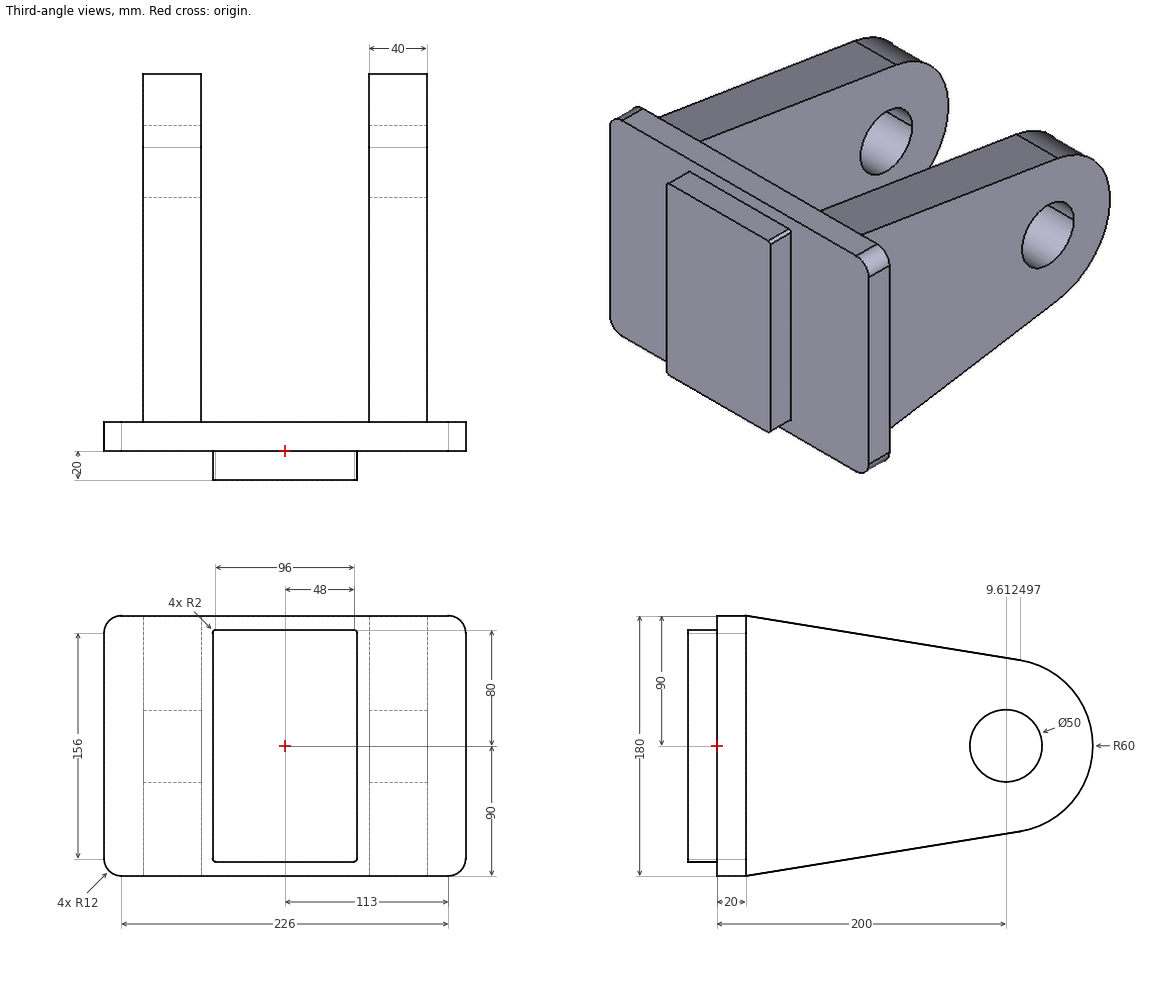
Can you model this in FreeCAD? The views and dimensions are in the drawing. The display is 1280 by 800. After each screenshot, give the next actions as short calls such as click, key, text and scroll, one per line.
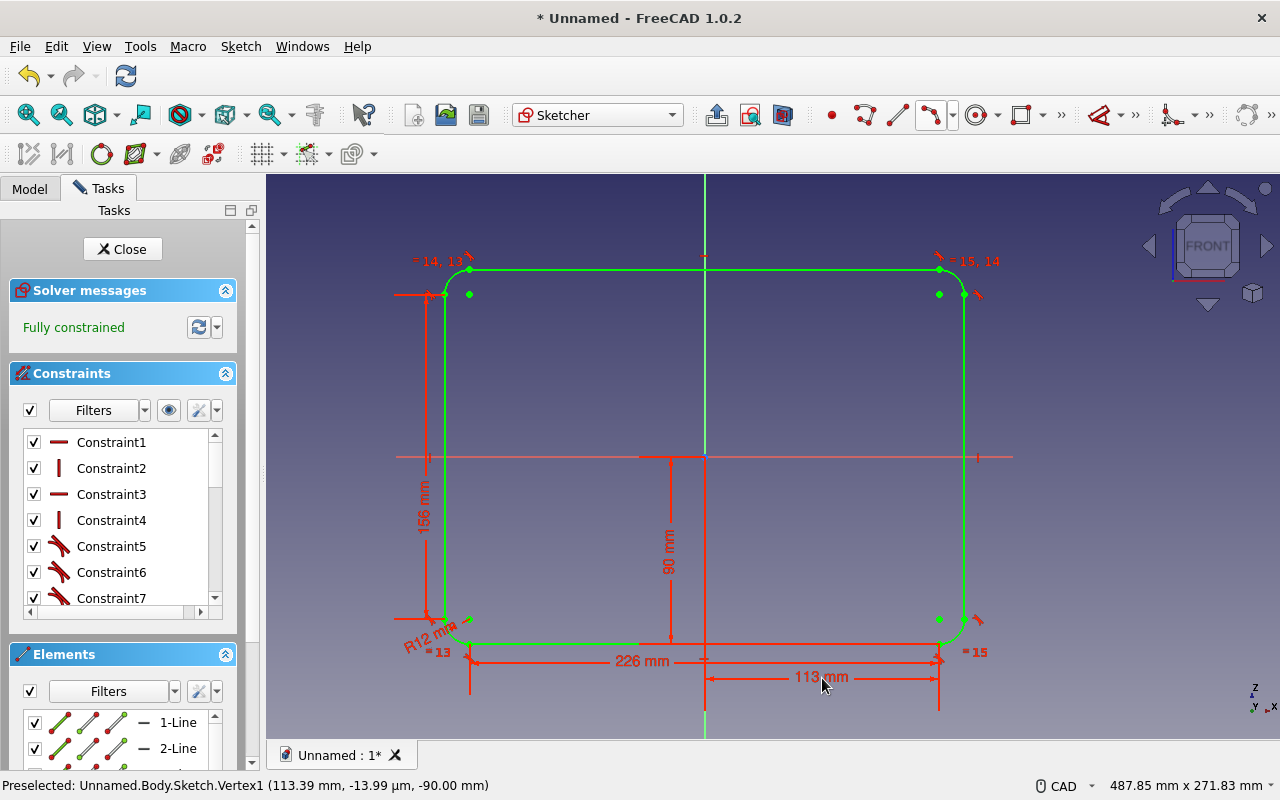
click(123, 249)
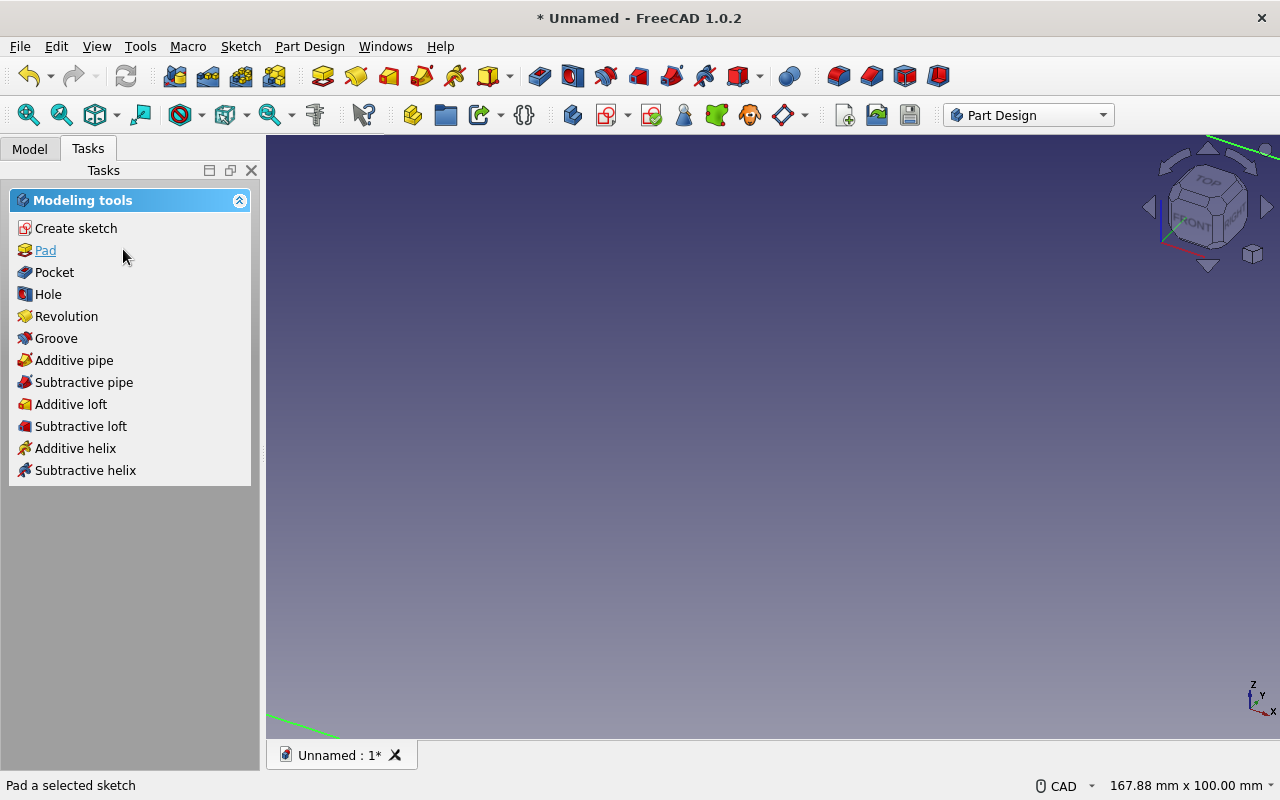
click(323, 76)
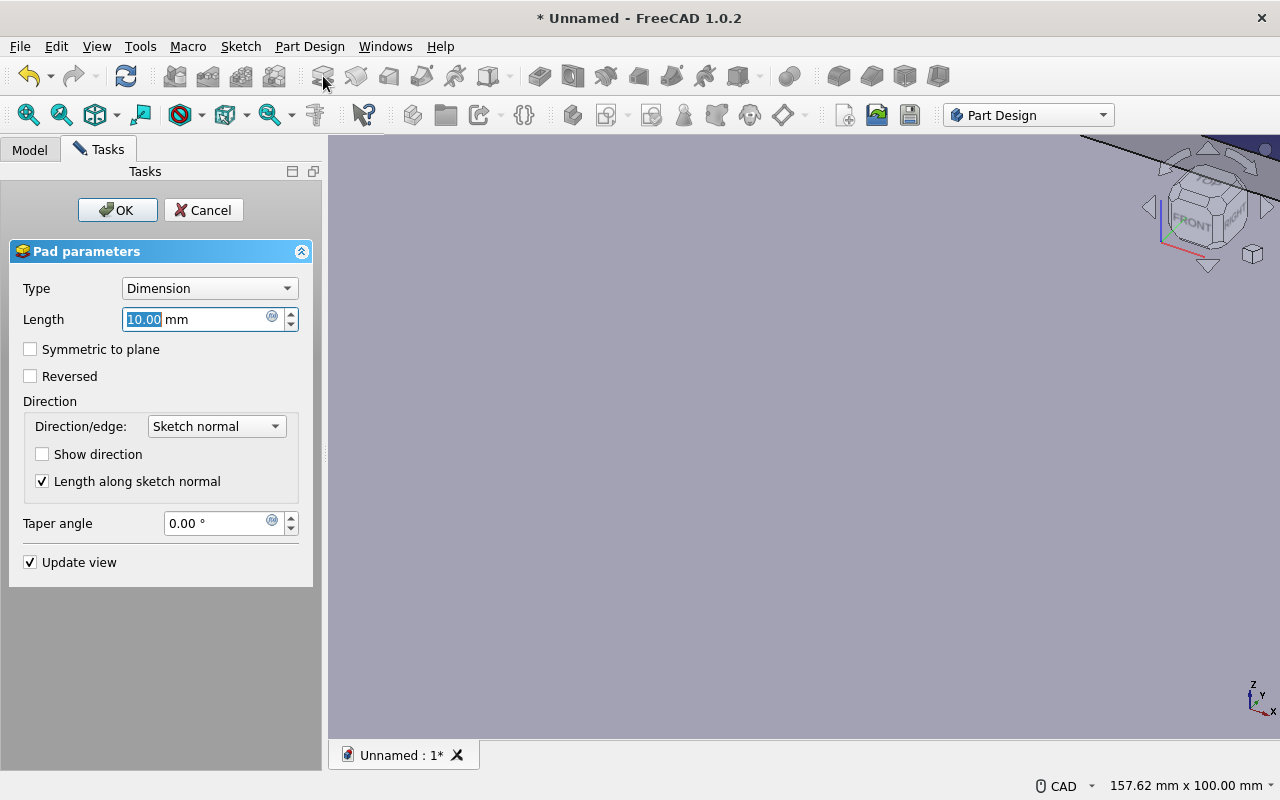
text(20)
key(Tab)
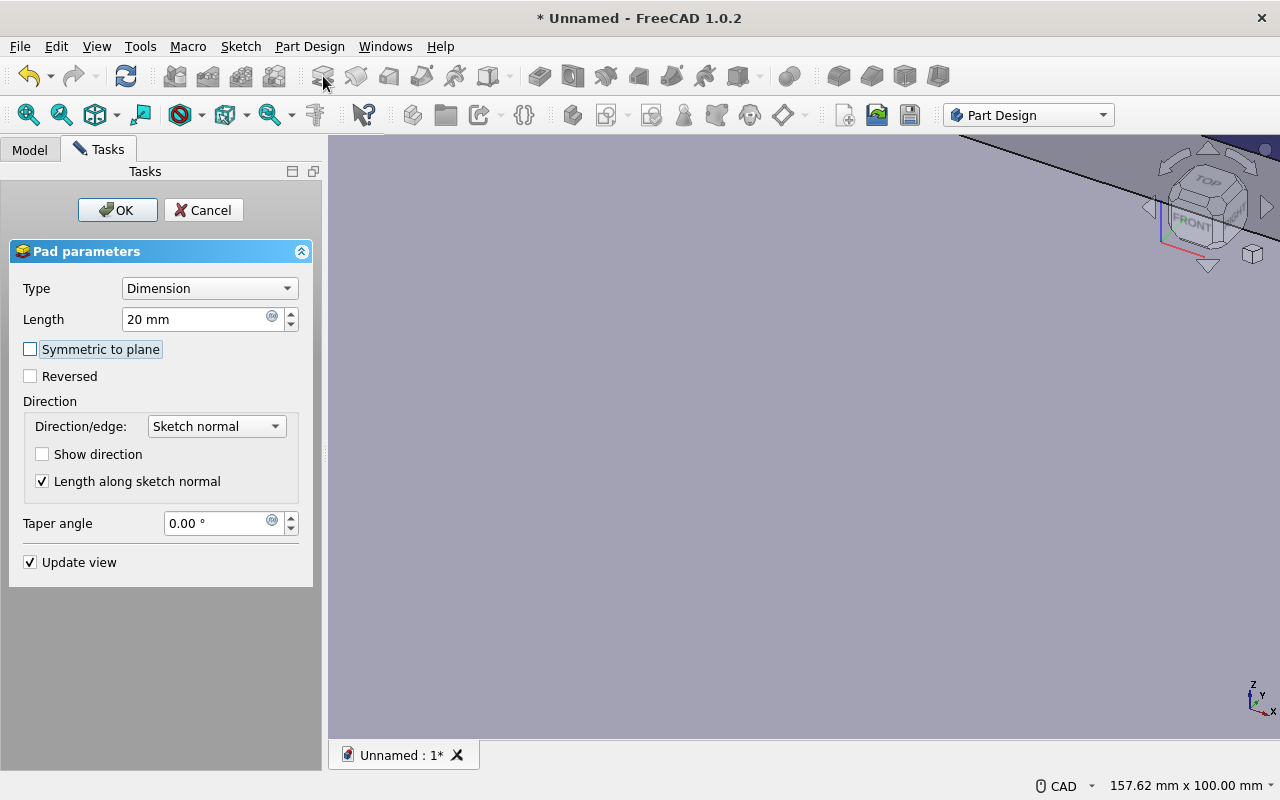
click(31, 376)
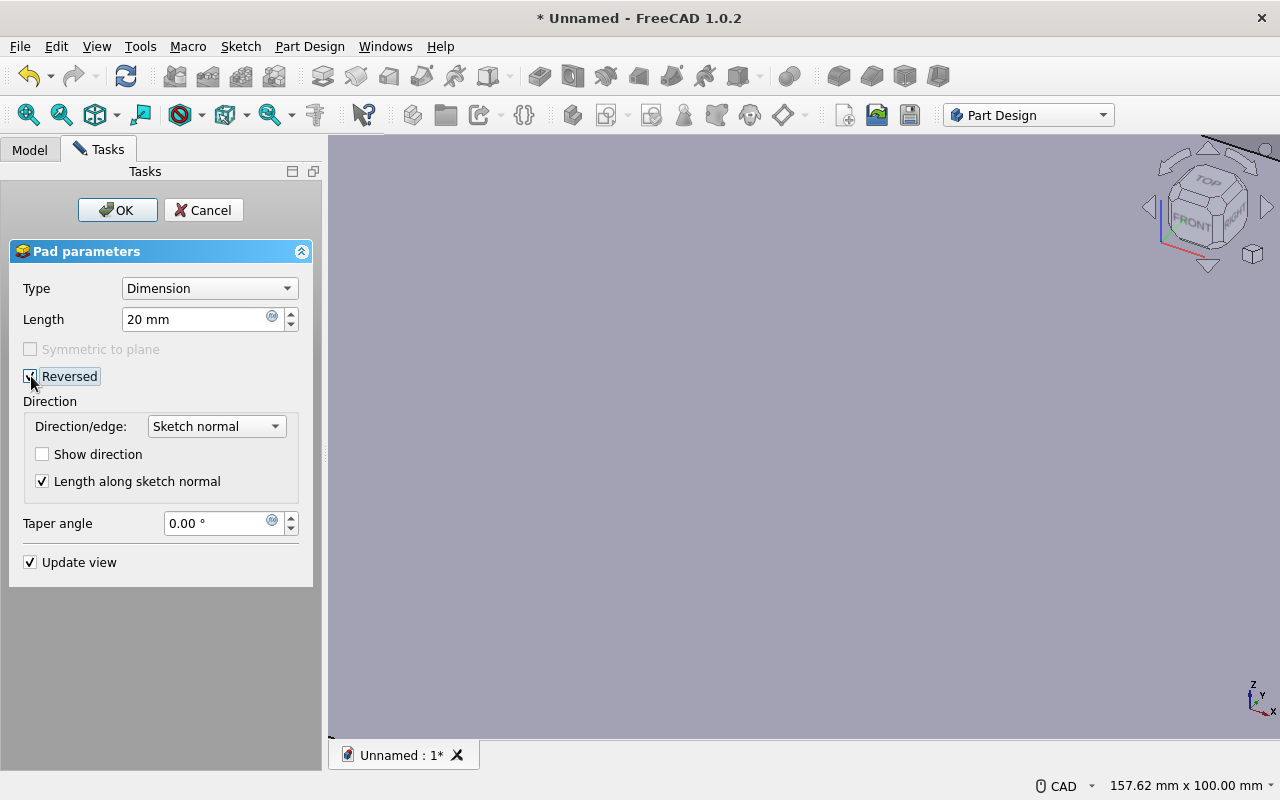
click(118, 210)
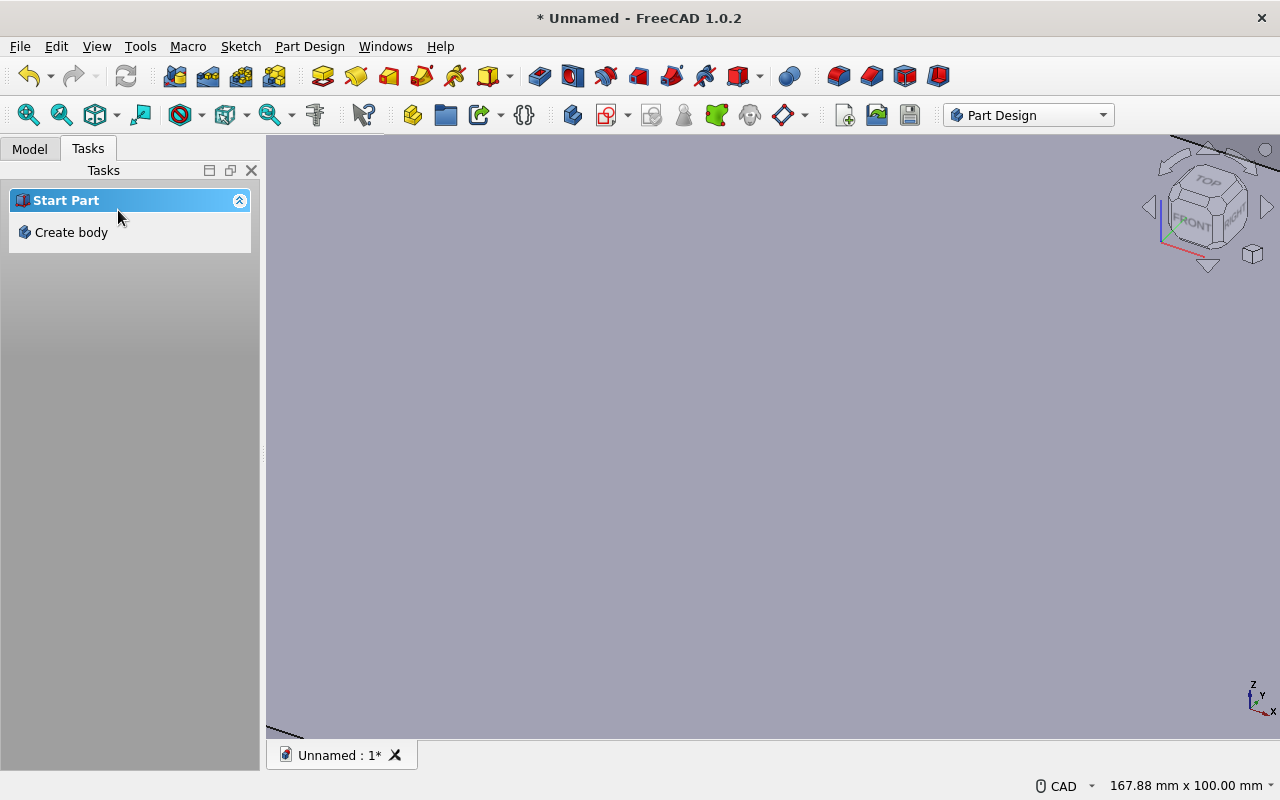
click(29, 116)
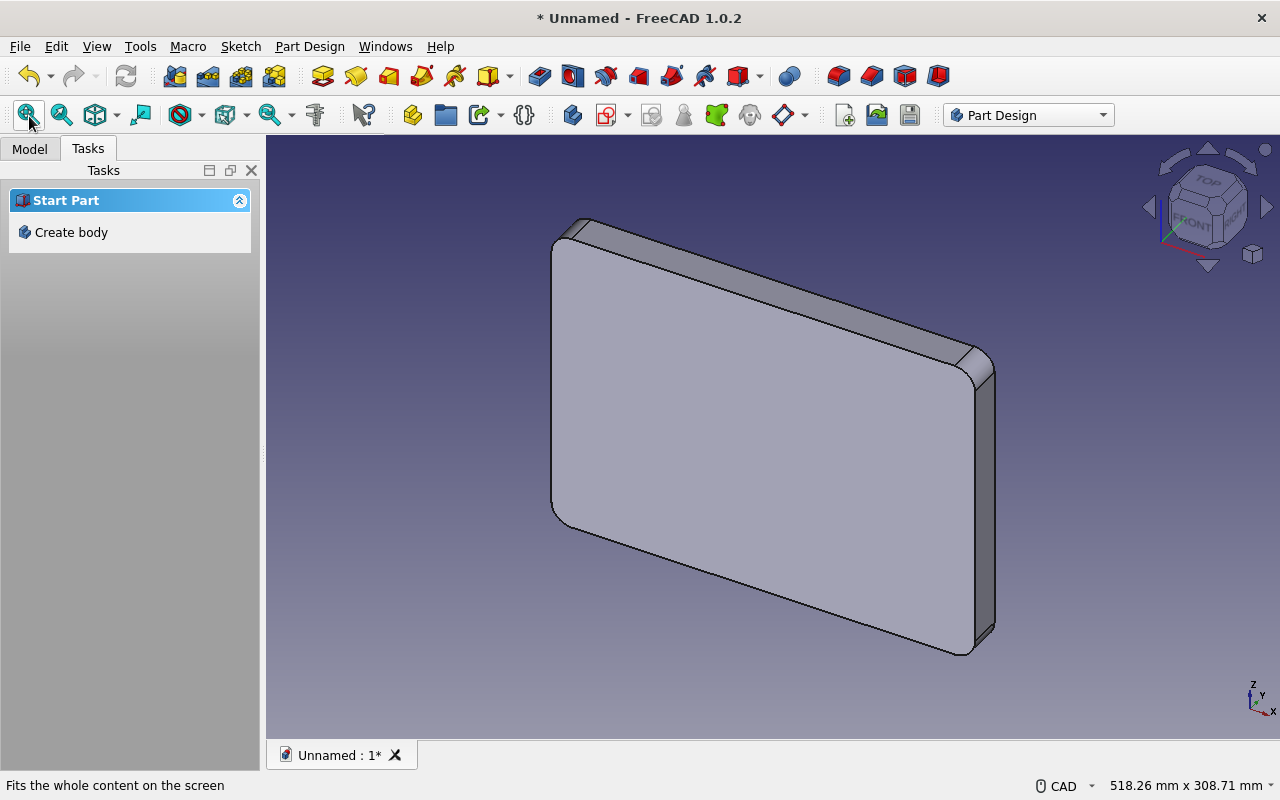
click(763, 446)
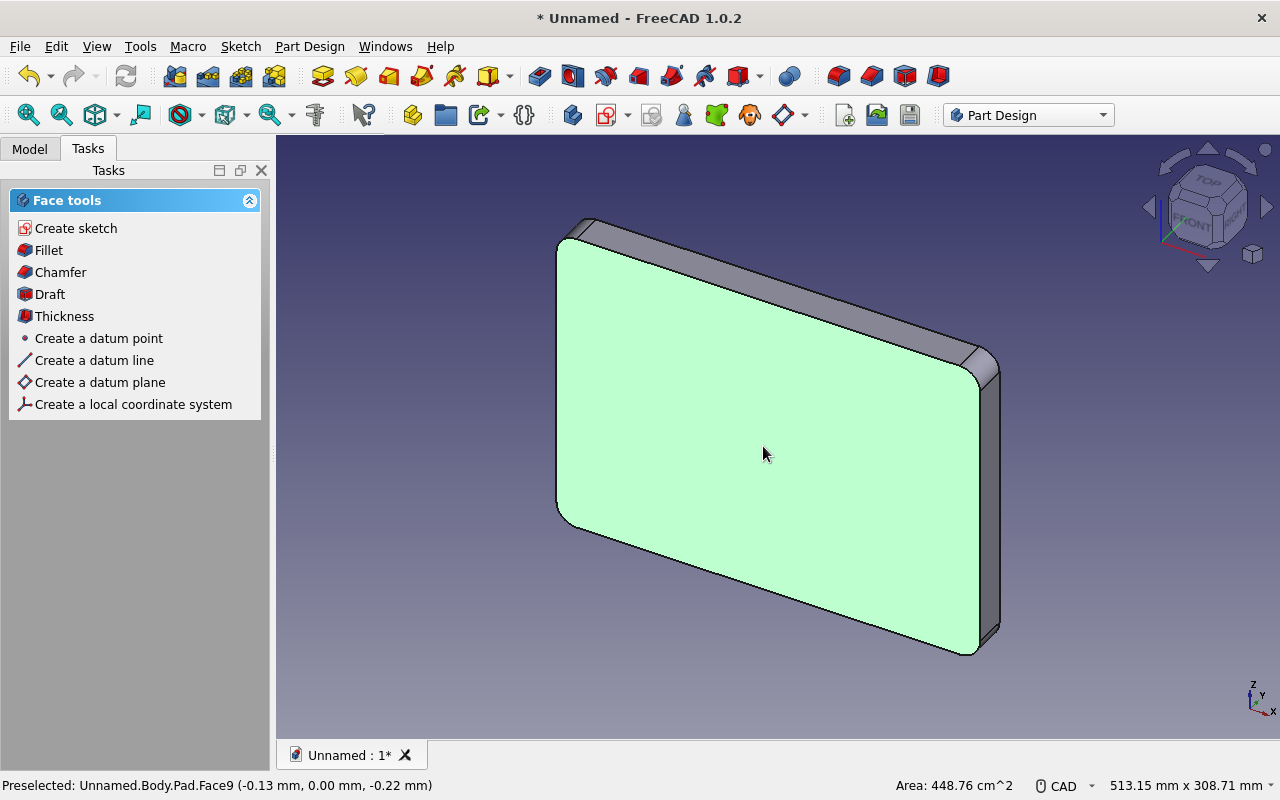
click(606, 116)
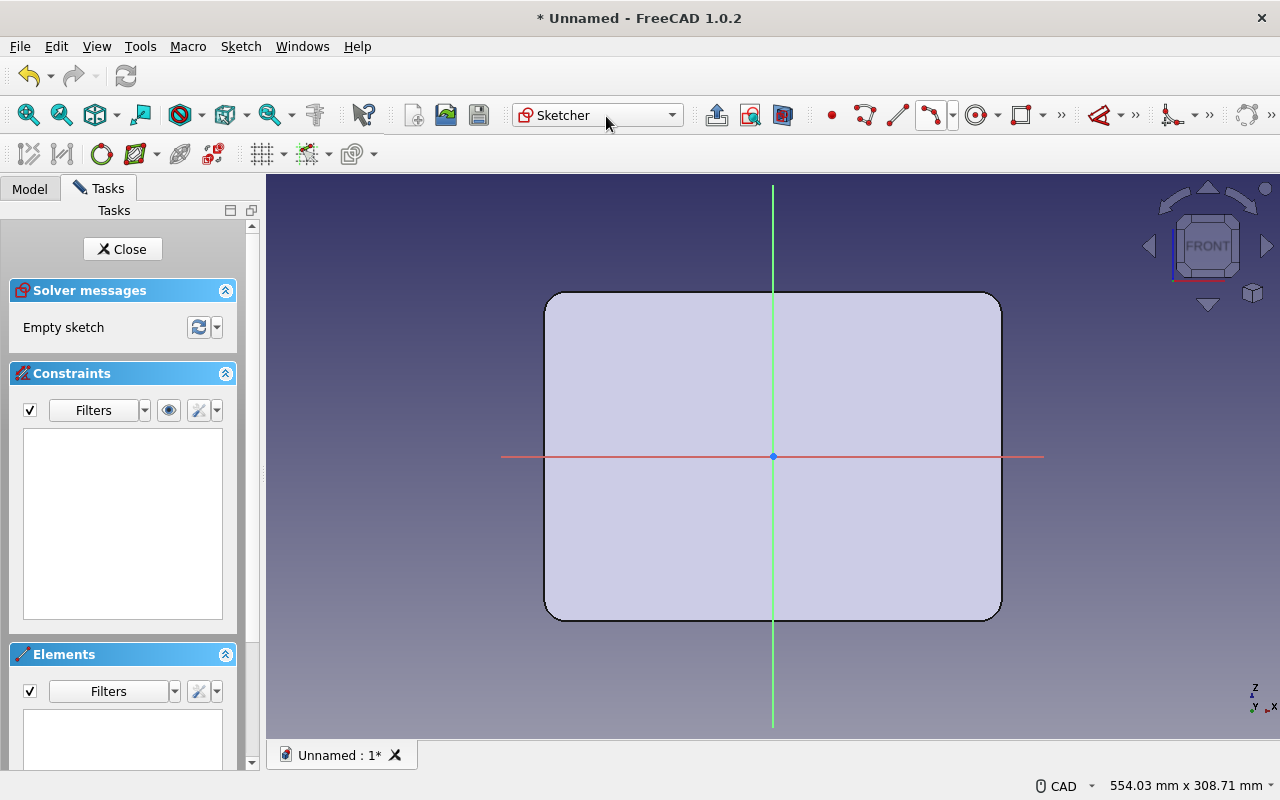
click(898, 116)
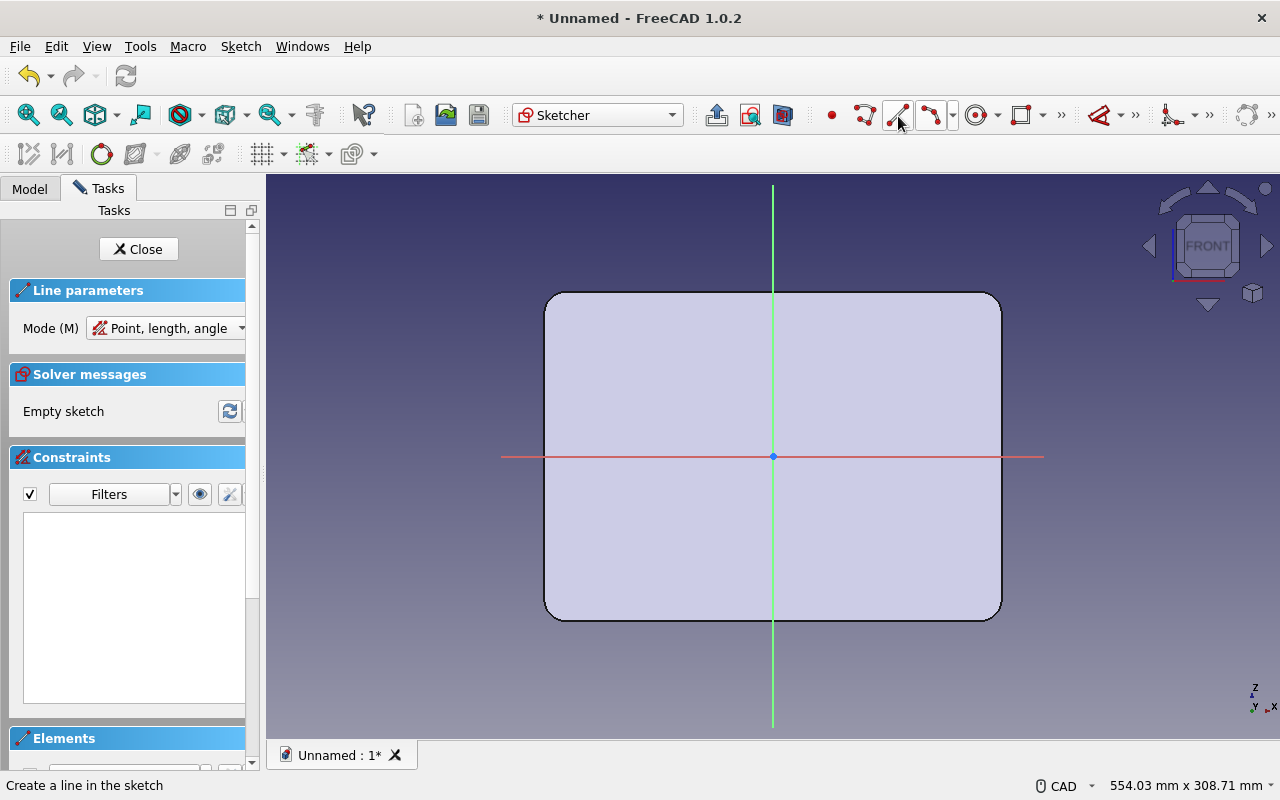
click(861, 310)
click(685, 310)